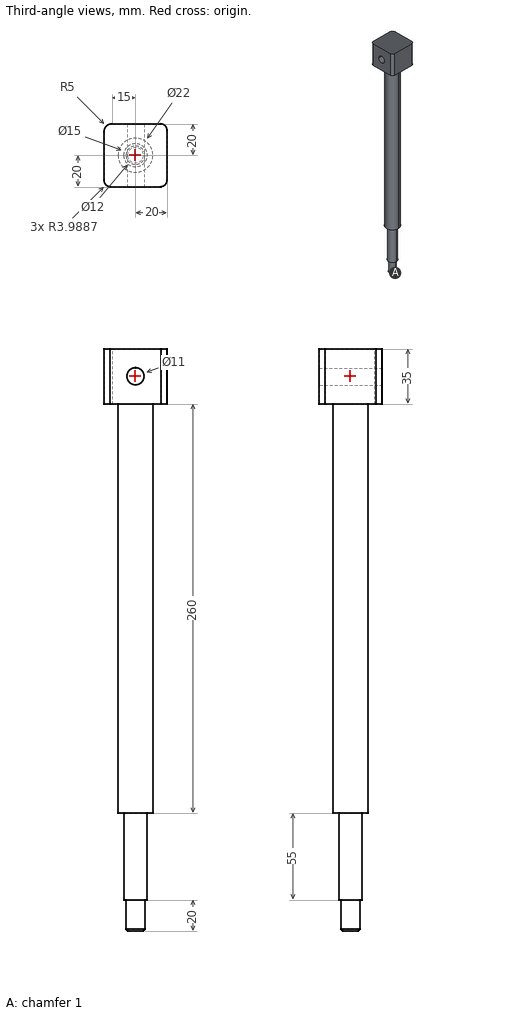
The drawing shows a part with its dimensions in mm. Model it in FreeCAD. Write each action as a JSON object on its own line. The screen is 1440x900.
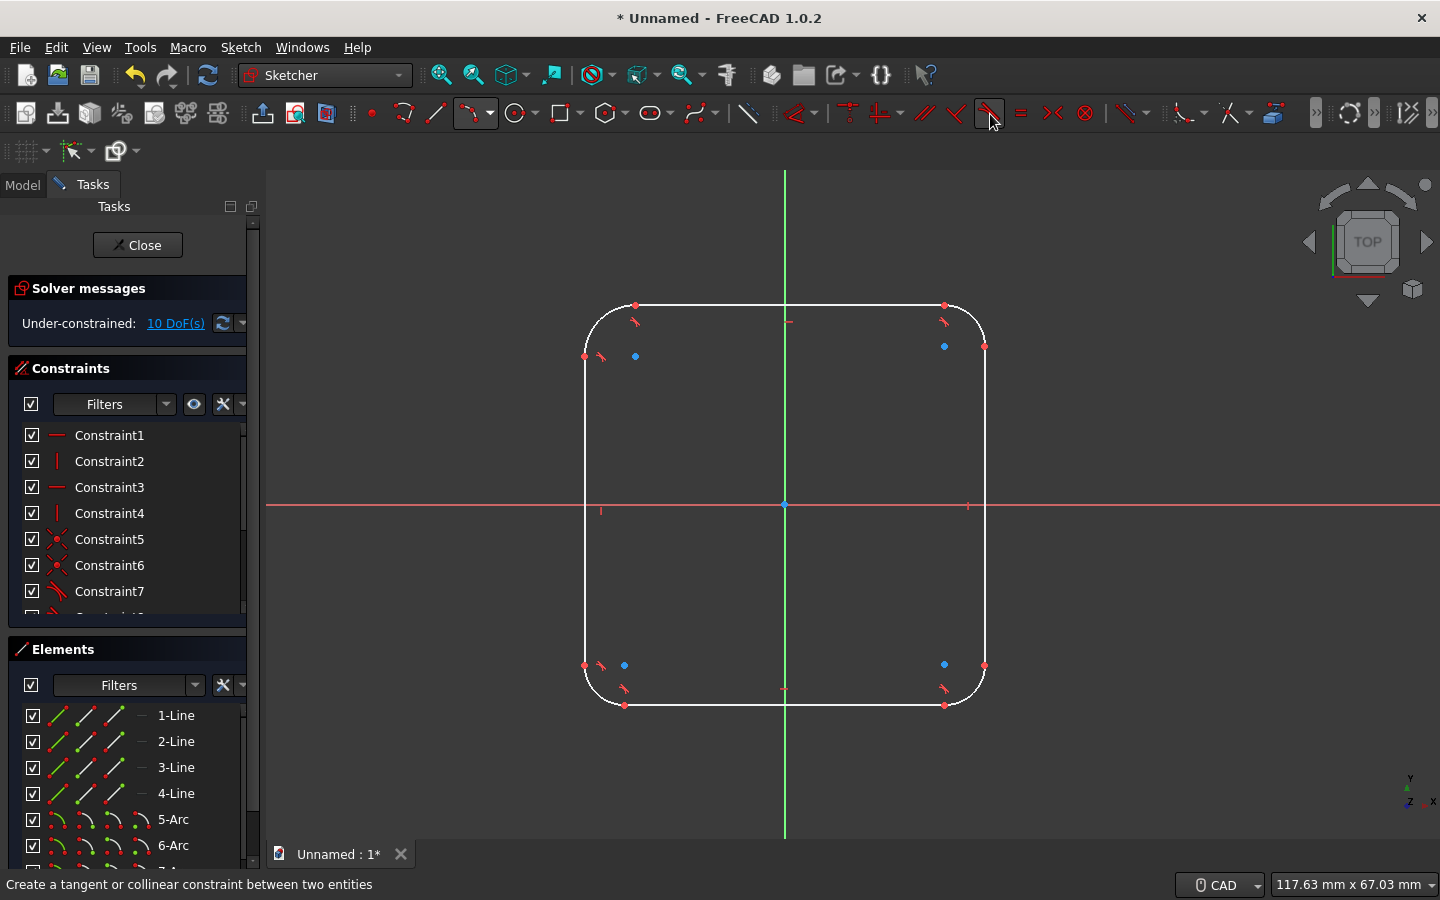
{"action": "left_click", "coordinate": [985, 569]}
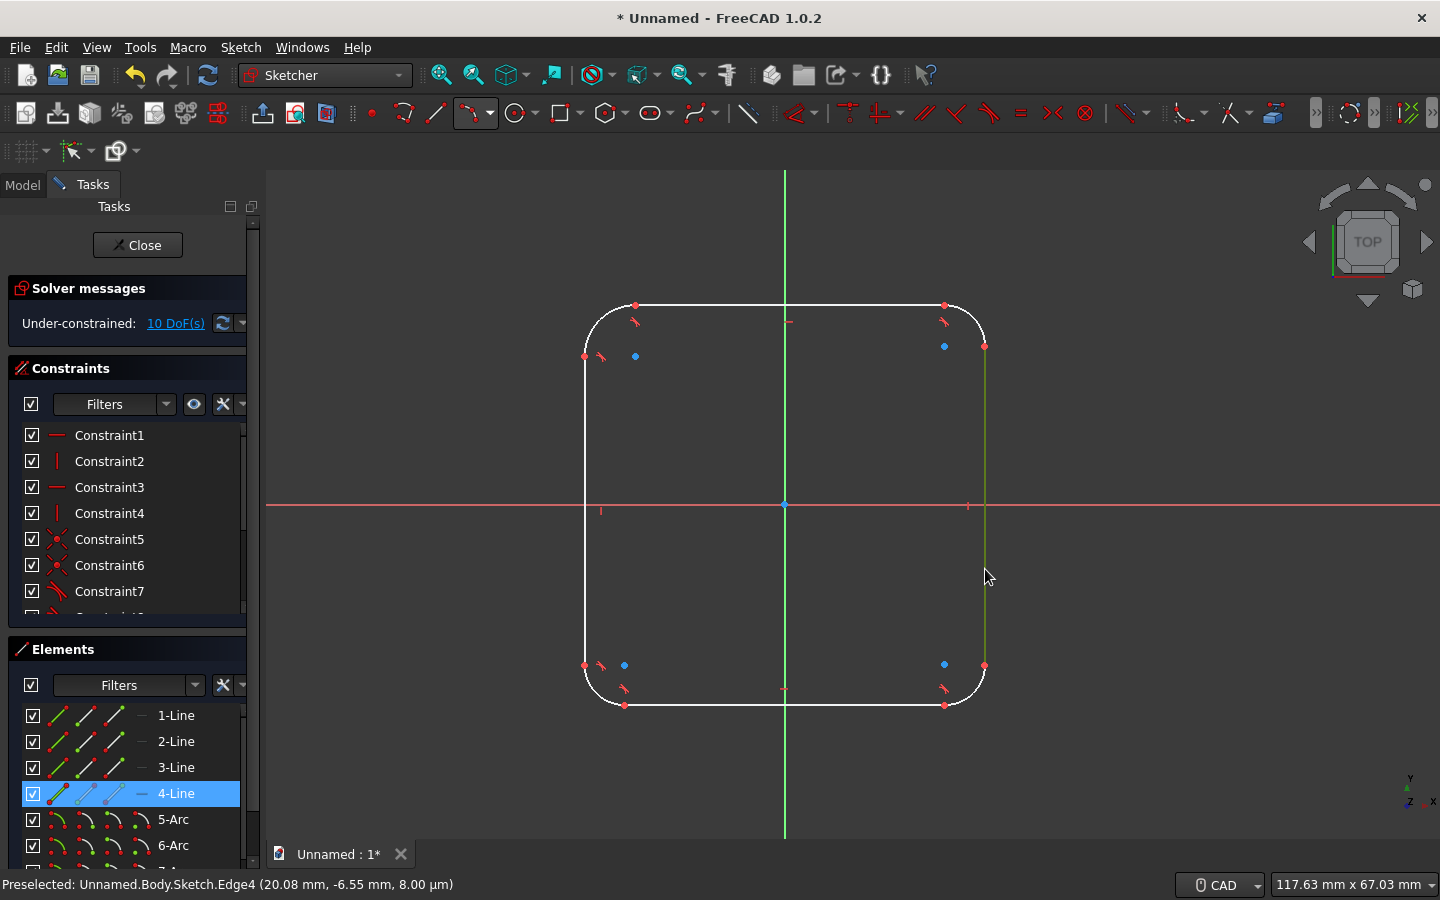
{"action": "left_click", "coordinate": [963, 701]}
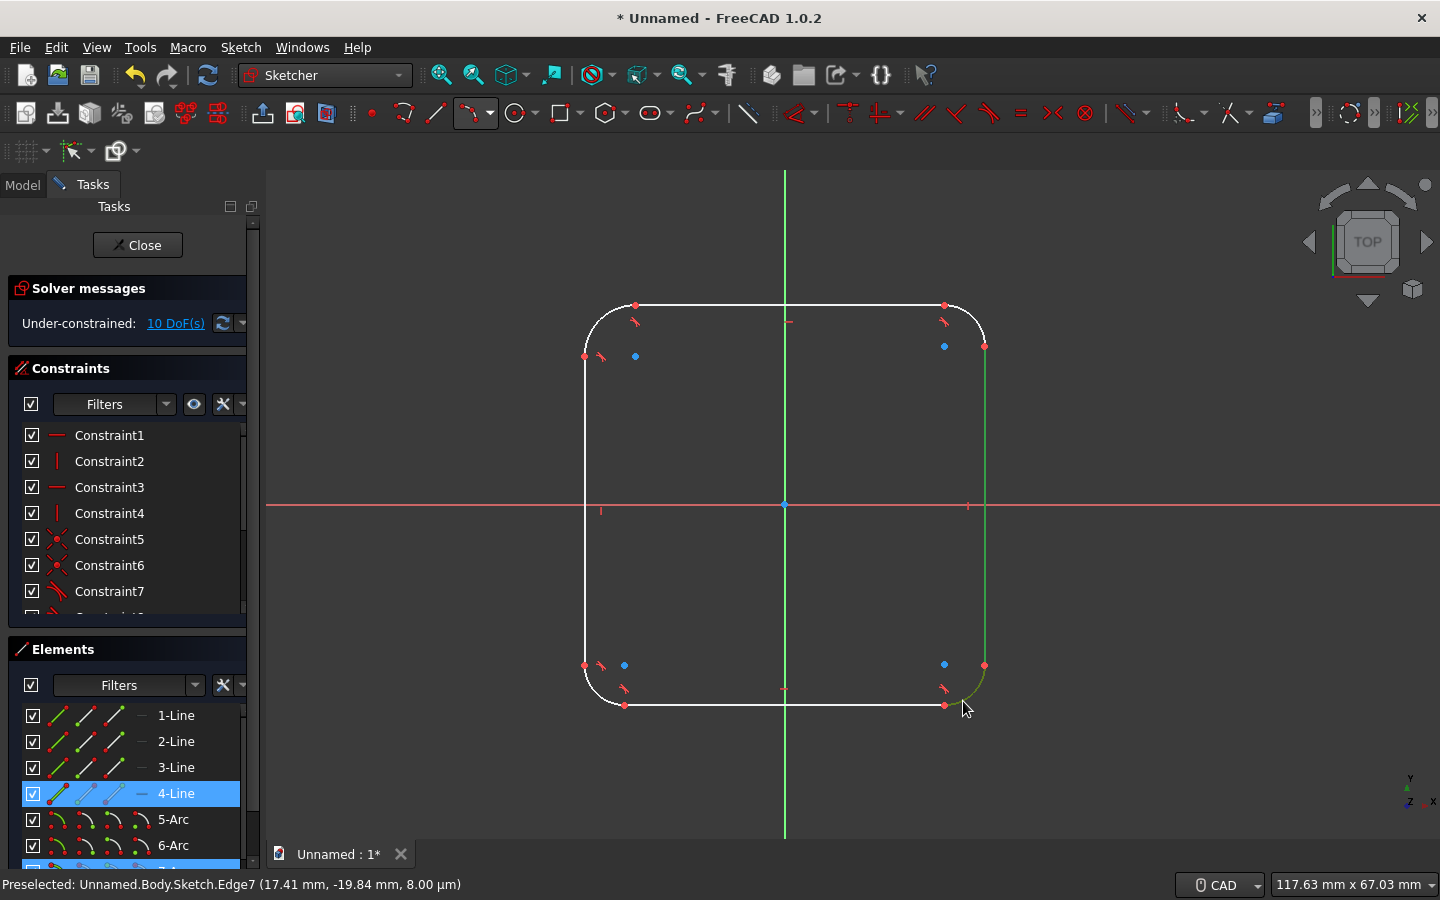
{"action": "left_click", "coordinate": [990, 114]}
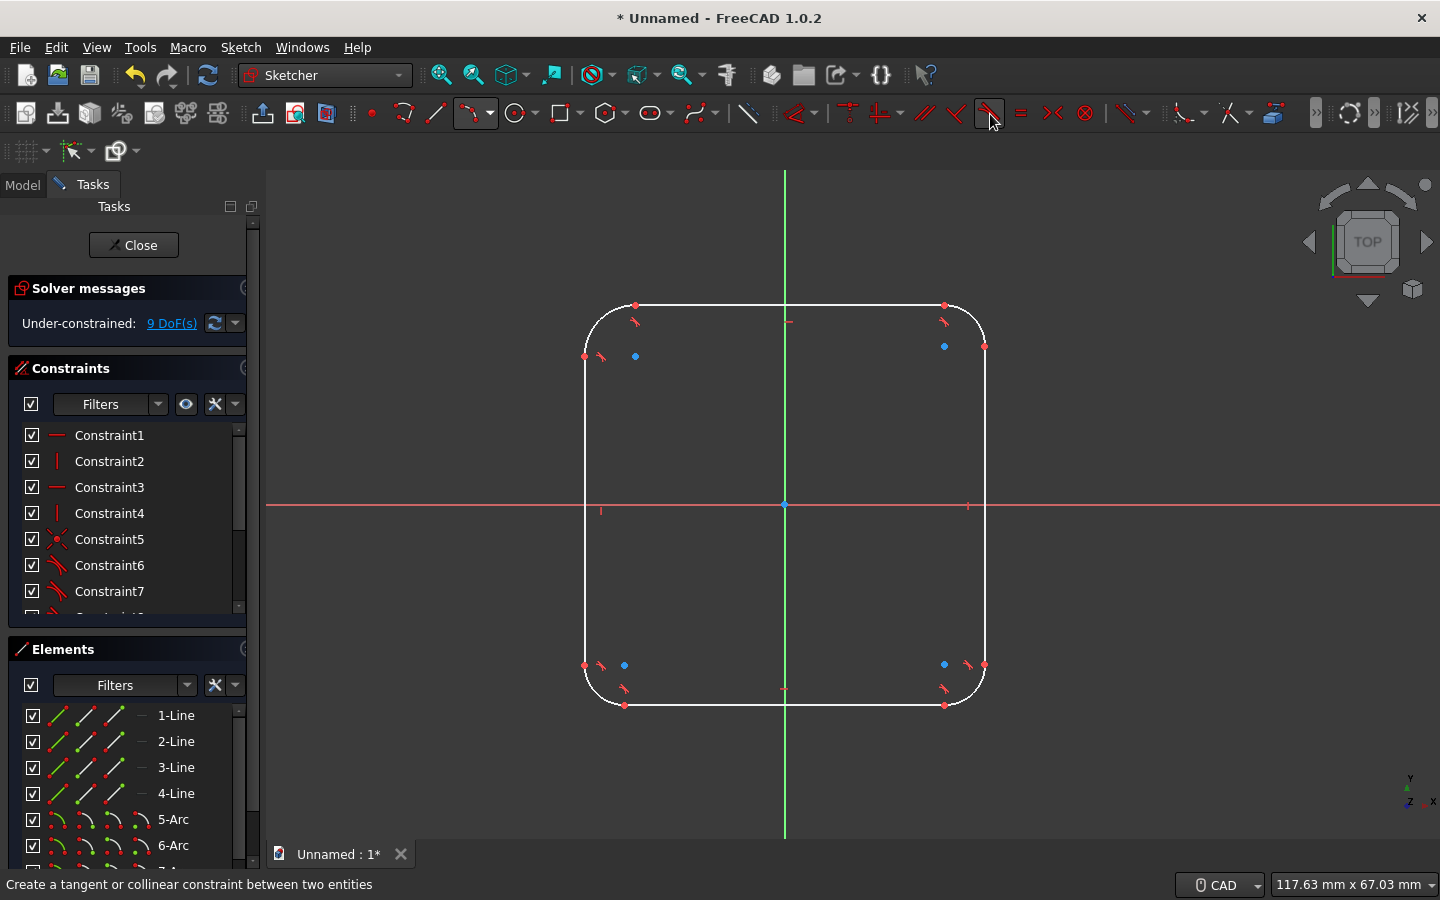
{"action": "left_click", "coordinate": [985, 569]}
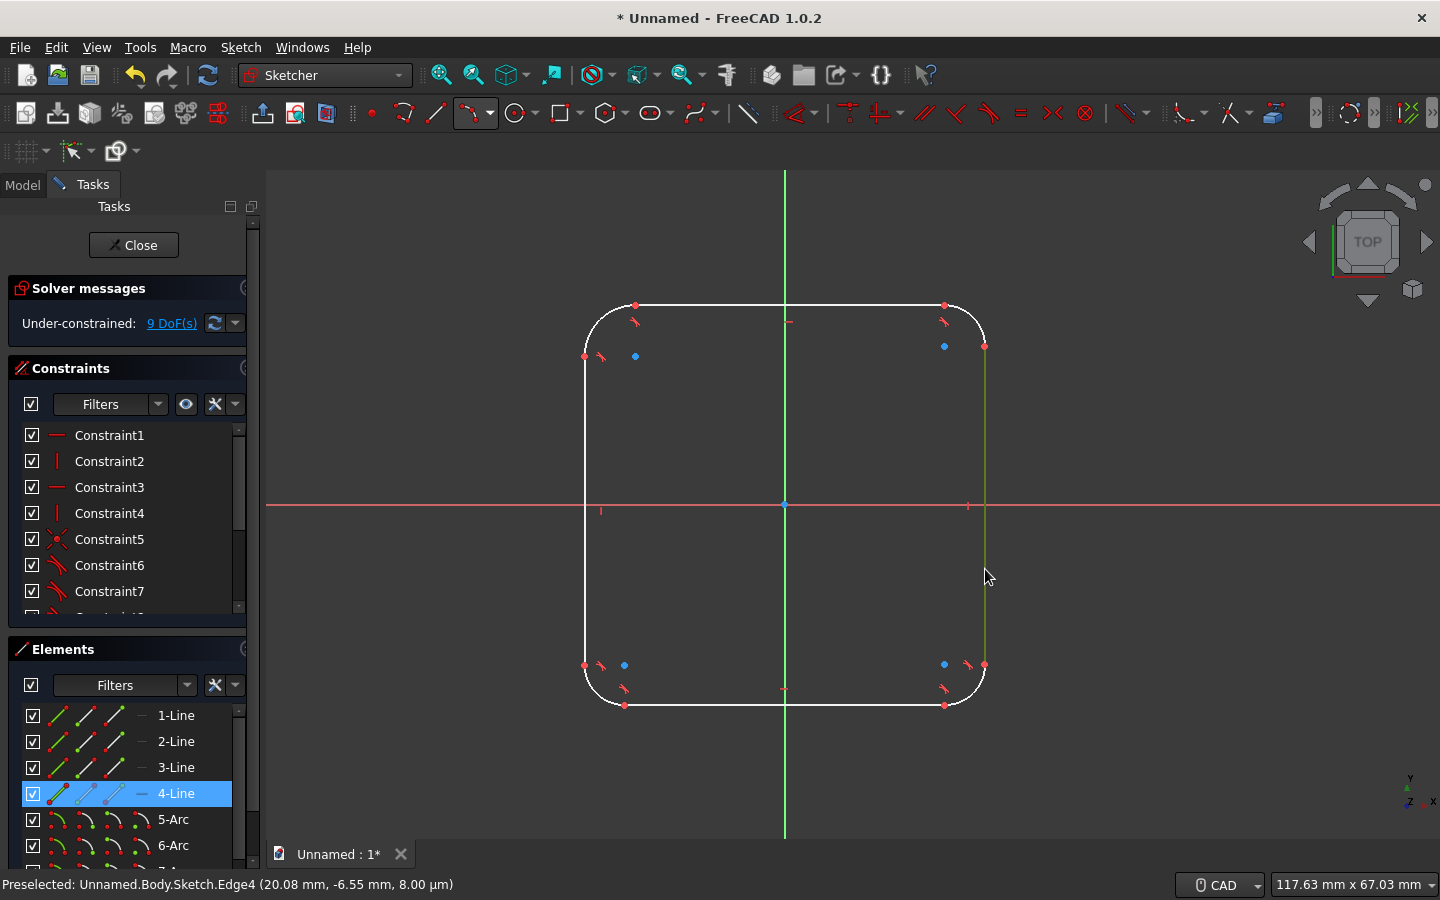
{"action": "left_click", "coordinate": [981, 328]}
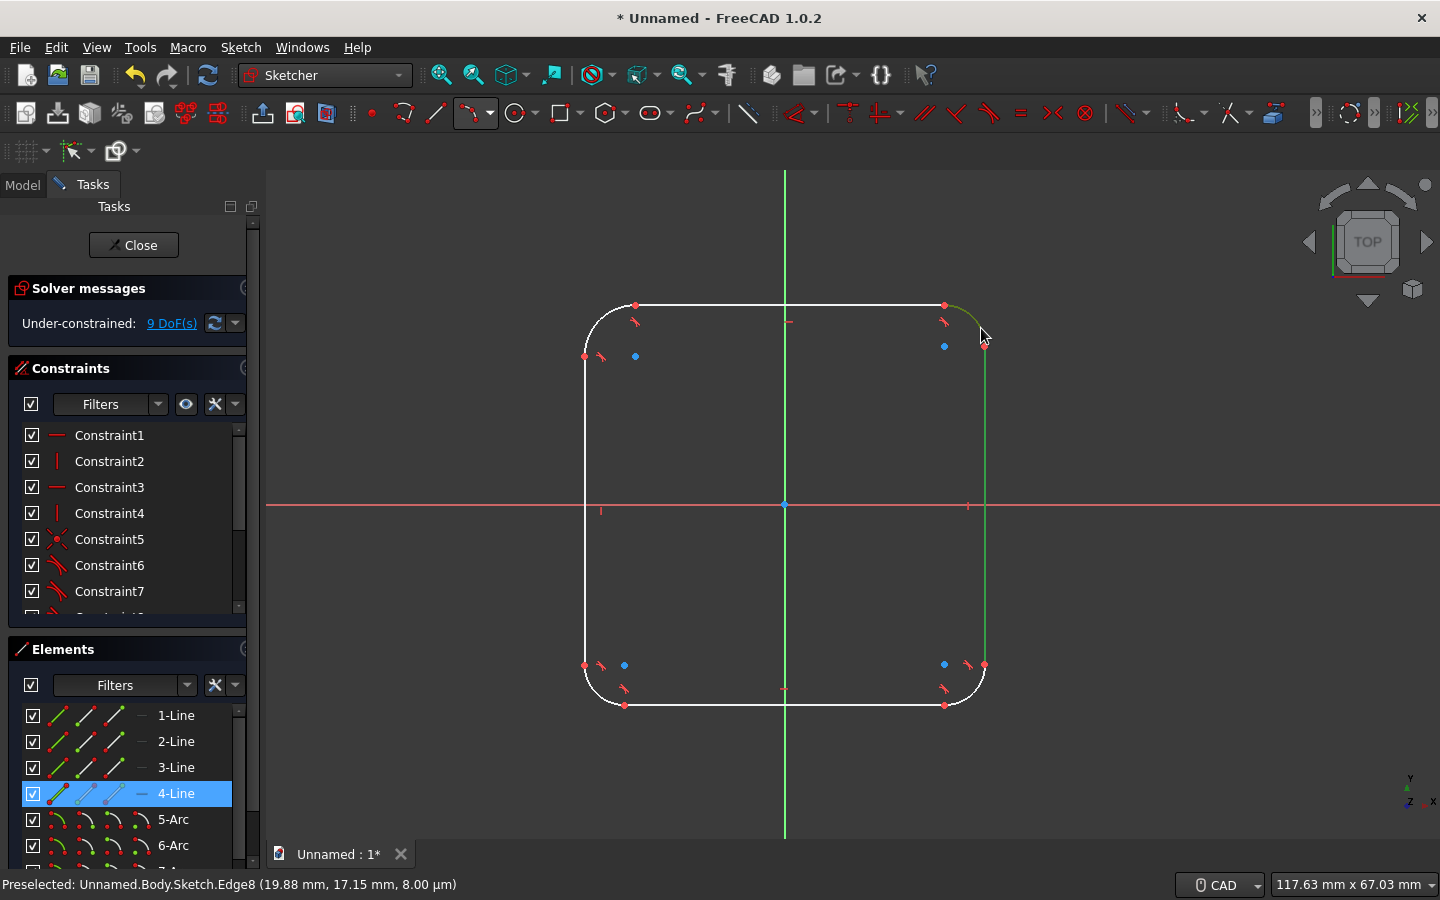
{"action": "left_click", "coordinate": [990, 114]}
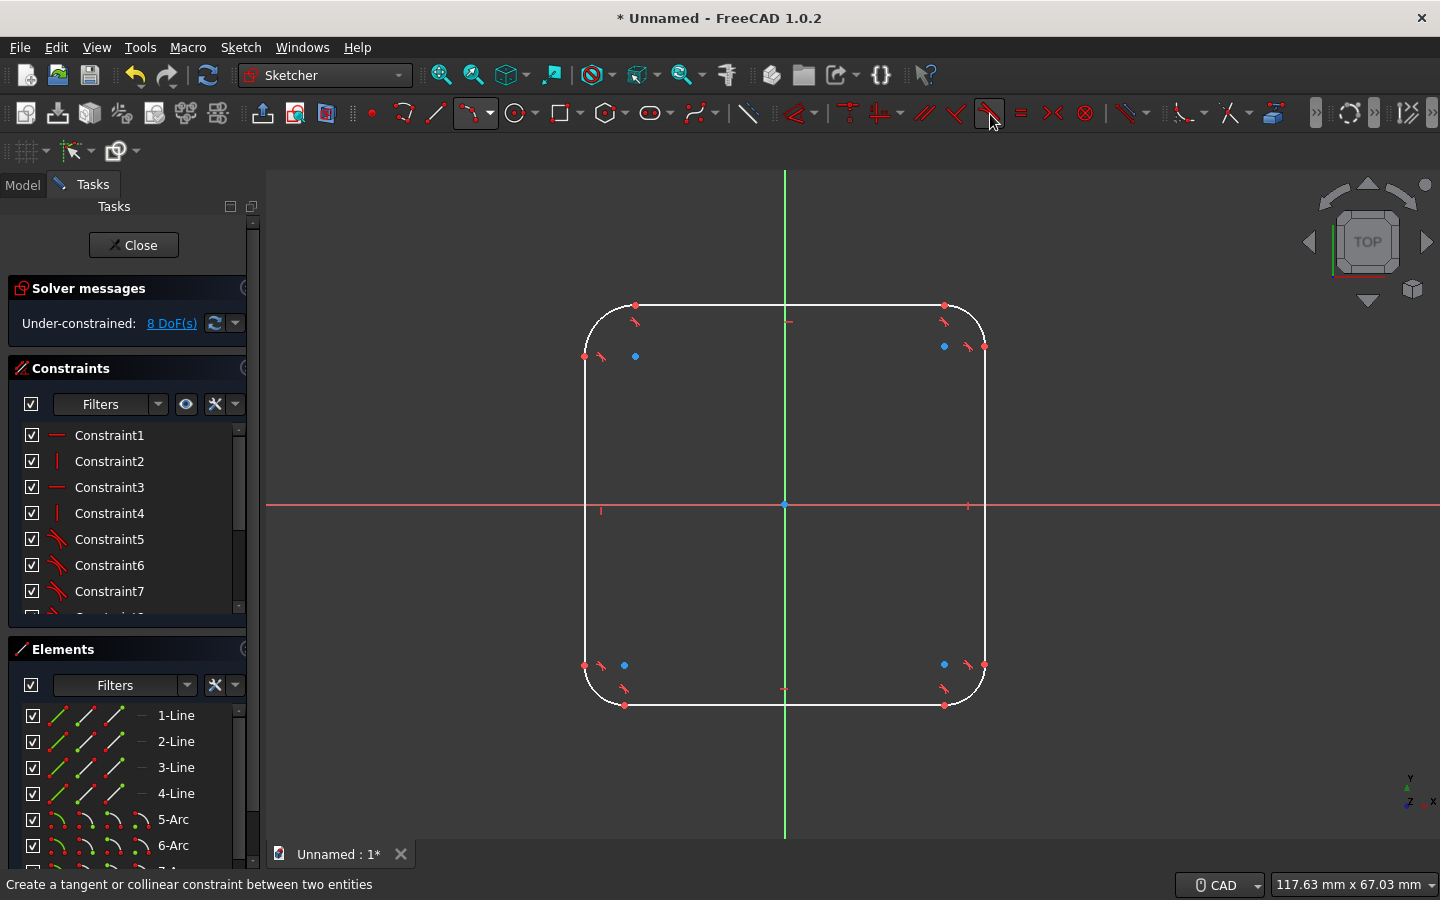
{"action": "left_click", "coordinate": [589, 683]}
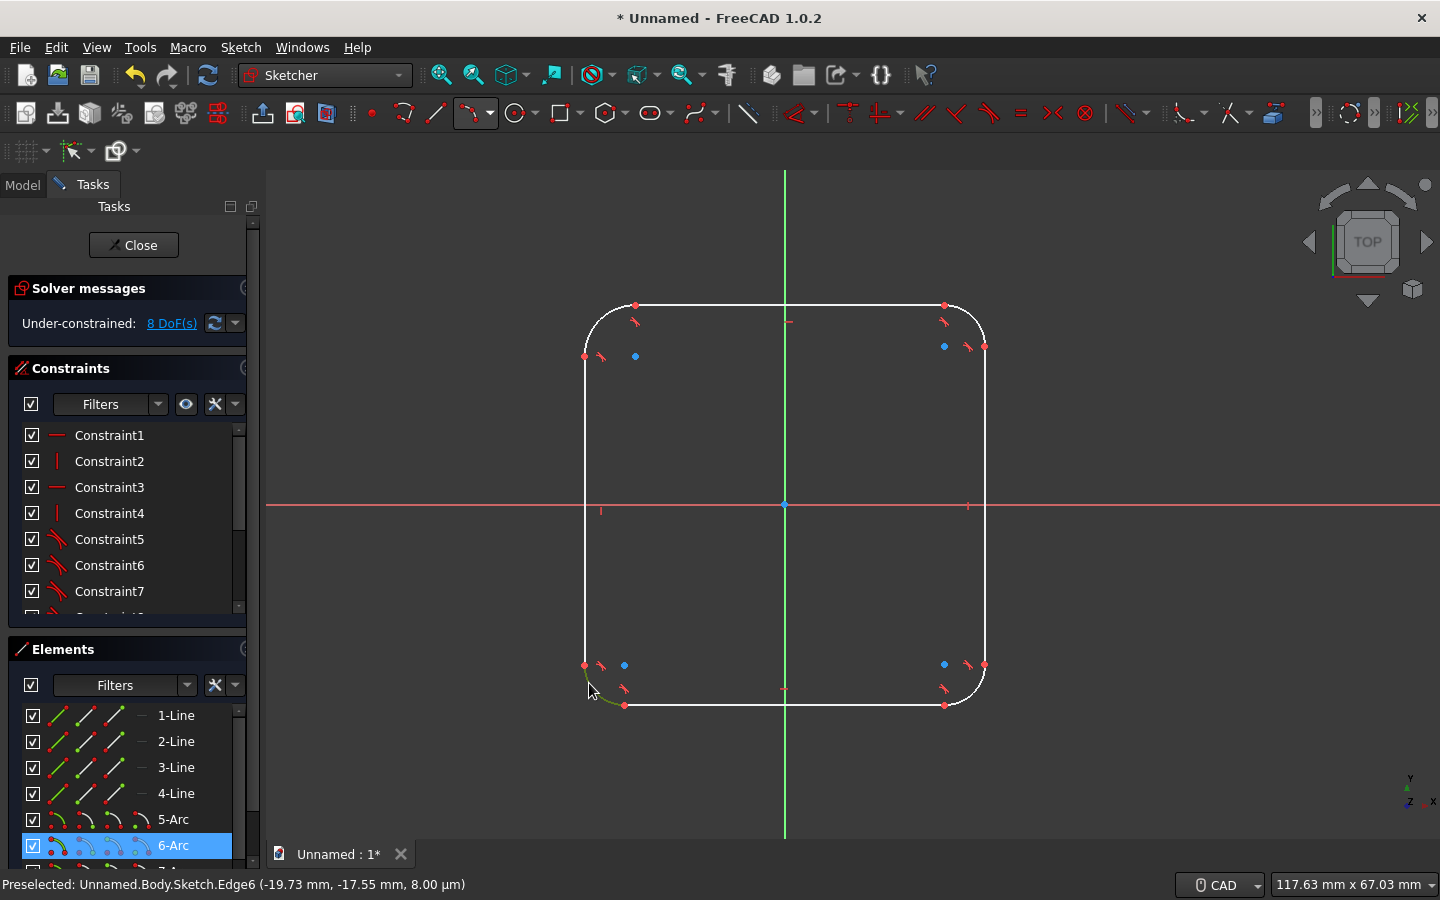
{"action": "left_click", "coordinate": [963, 701]}